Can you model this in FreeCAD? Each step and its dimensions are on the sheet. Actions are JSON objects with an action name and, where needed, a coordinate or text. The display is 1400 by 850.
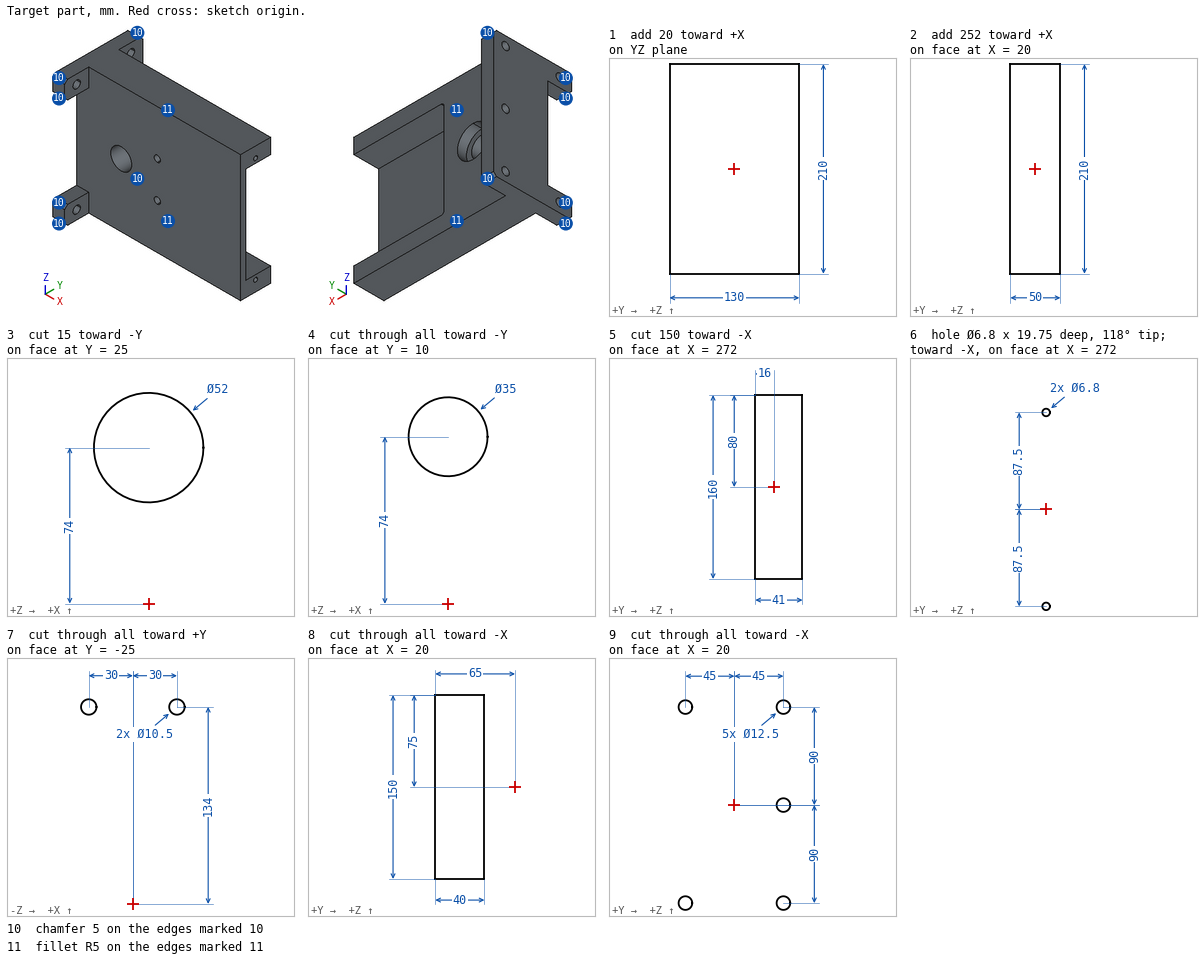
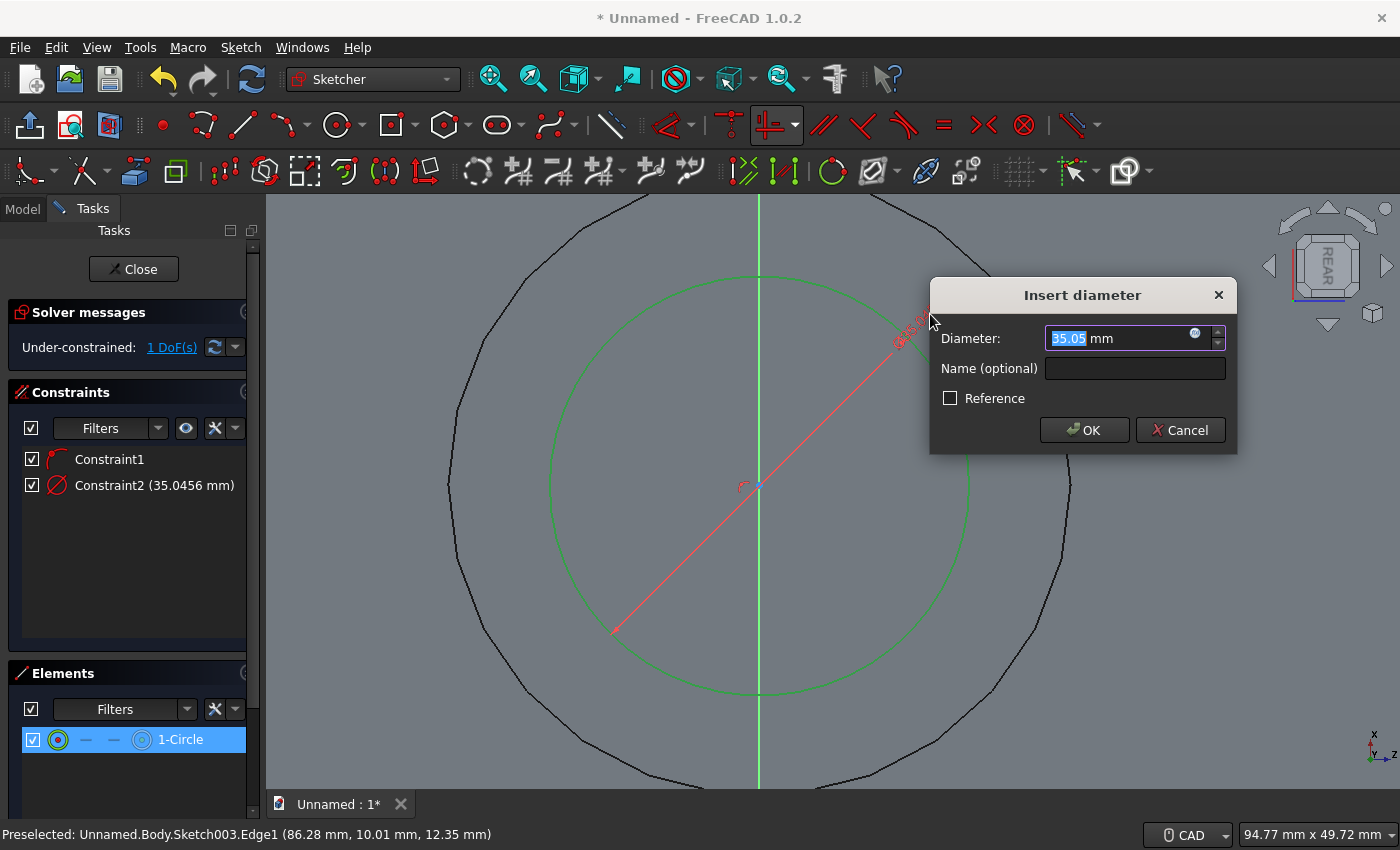
{"action": "type", "text": "35"}
{"action": "key", "text": "Return"}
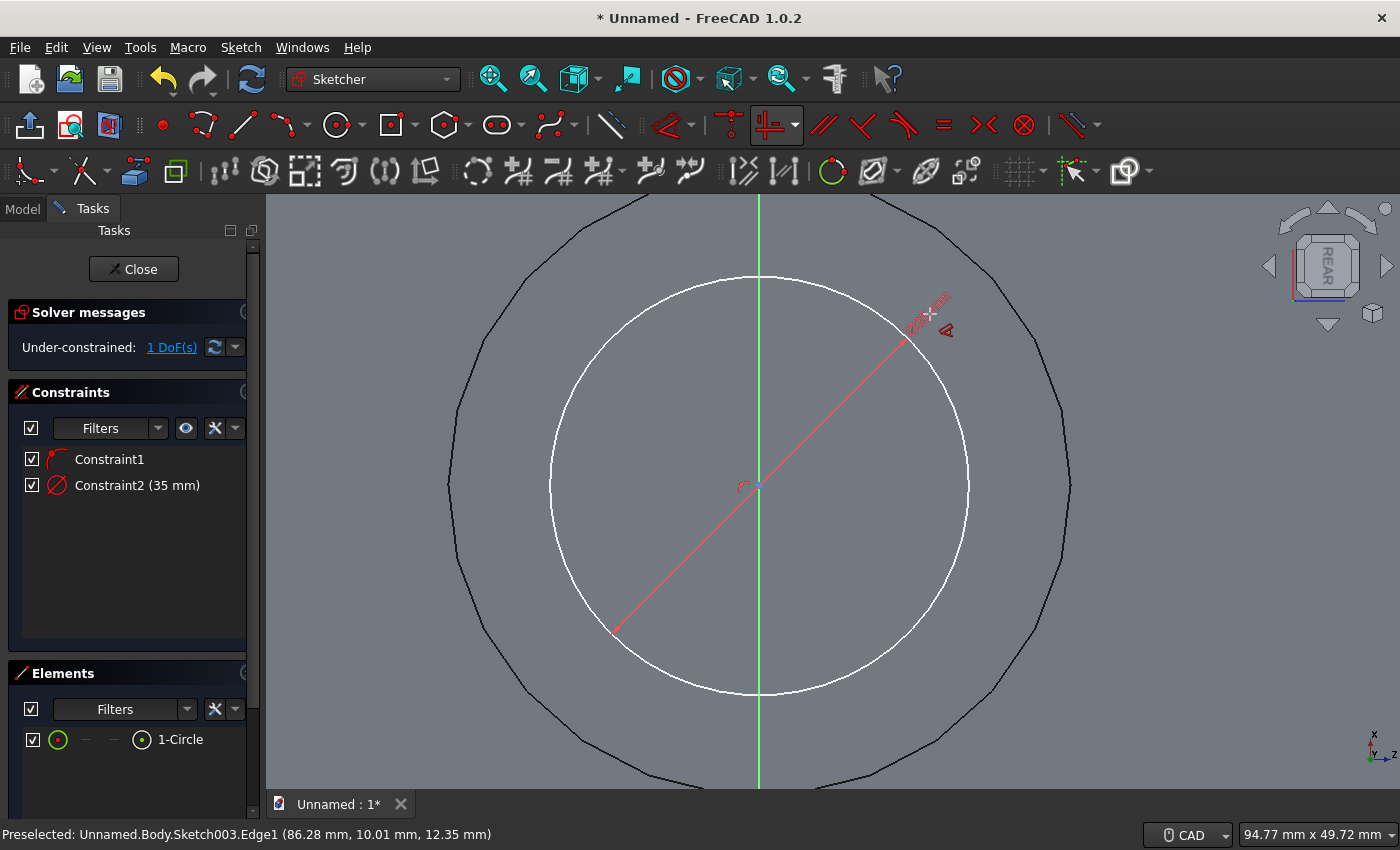
{"action": "left_click", "coordinate": [759, 486]}
{"action": "left_click", "coordinate": [793, 624]}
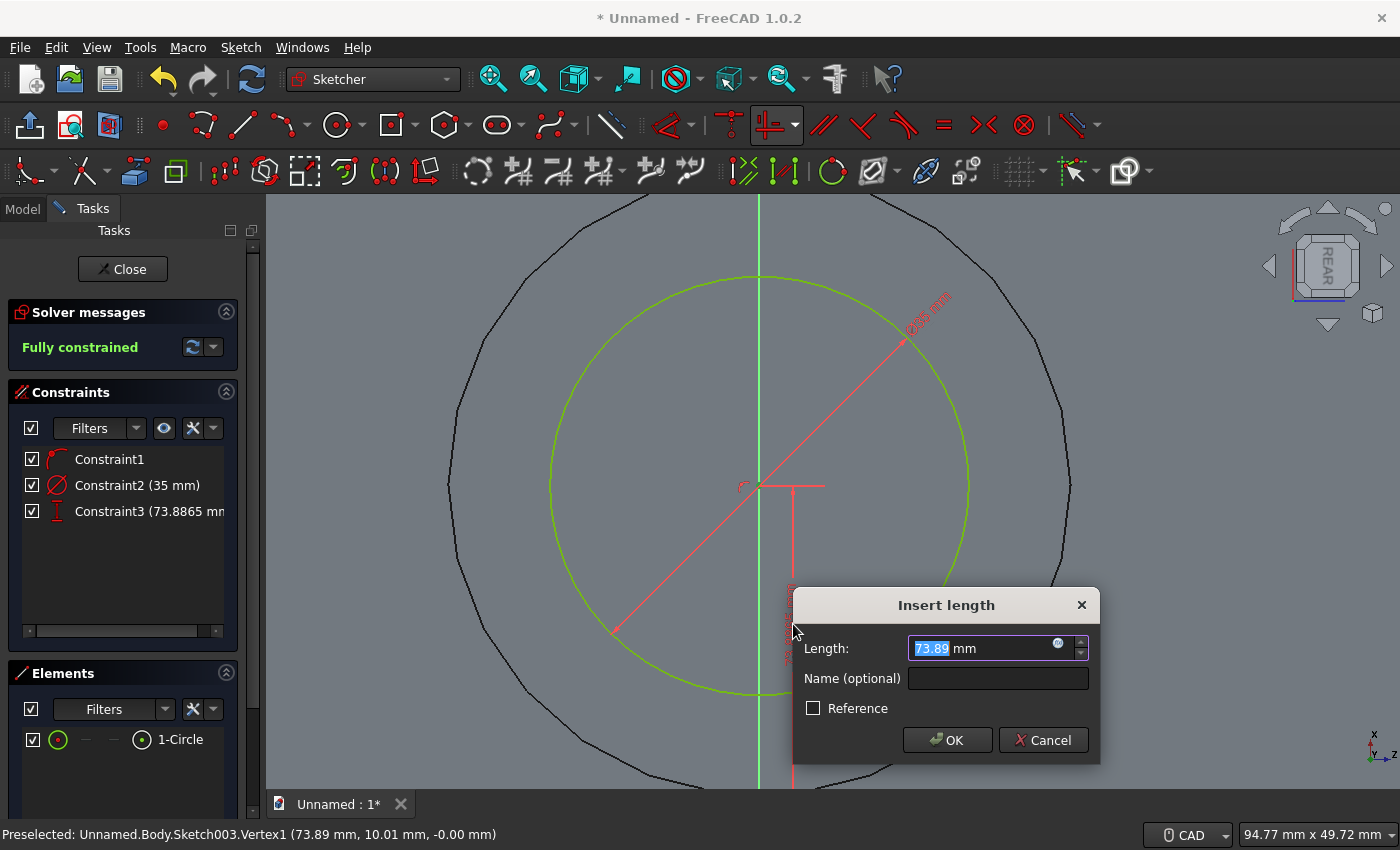
{"action": "type", "text": "74"}
{"action": "key", "text": "Return"}
{"action": "key", "text": "Escape"}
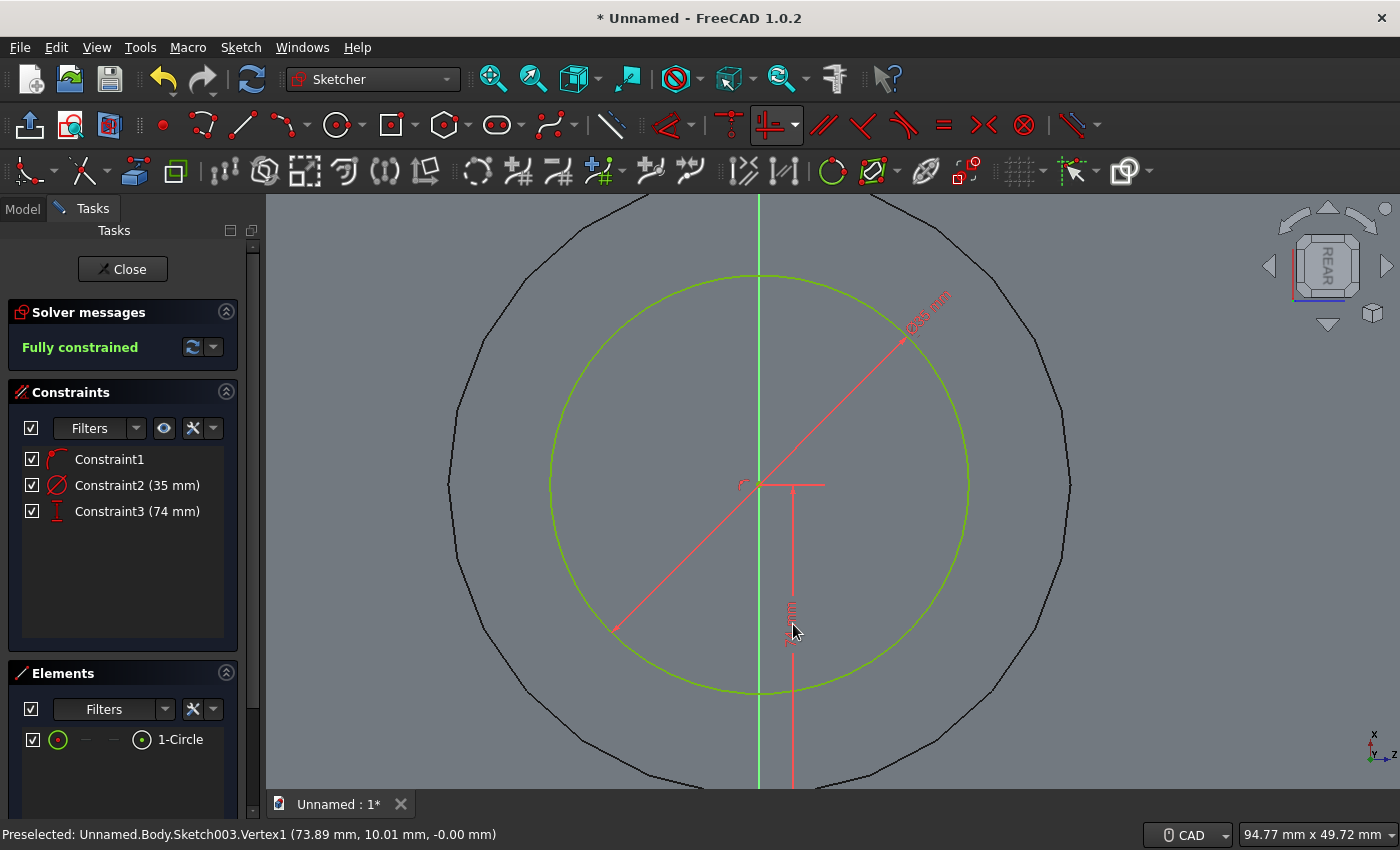
{"action": "left_click", "coordinate": [123, 269]}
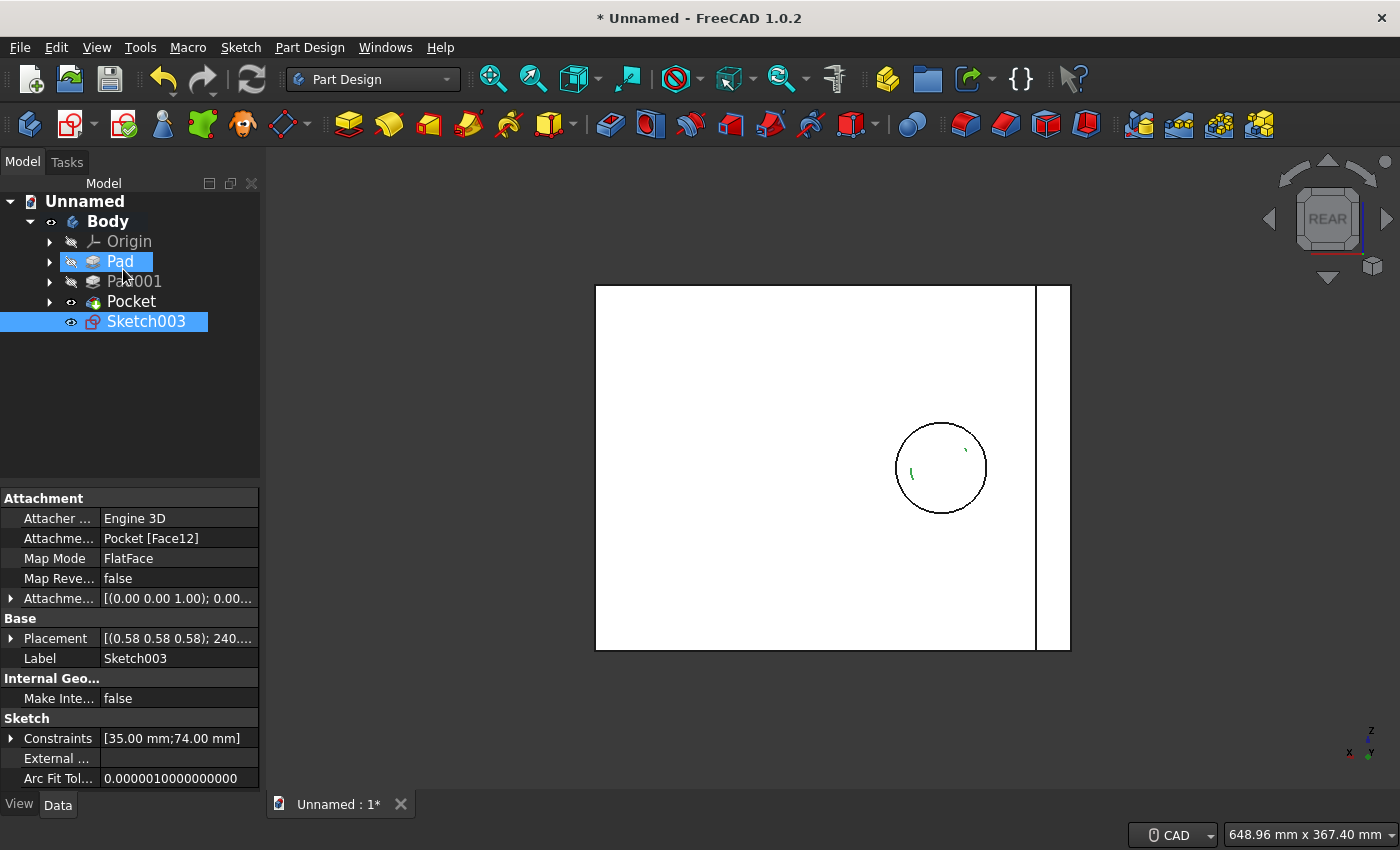
{"action": "left_click", "coordinate": [612, 124]}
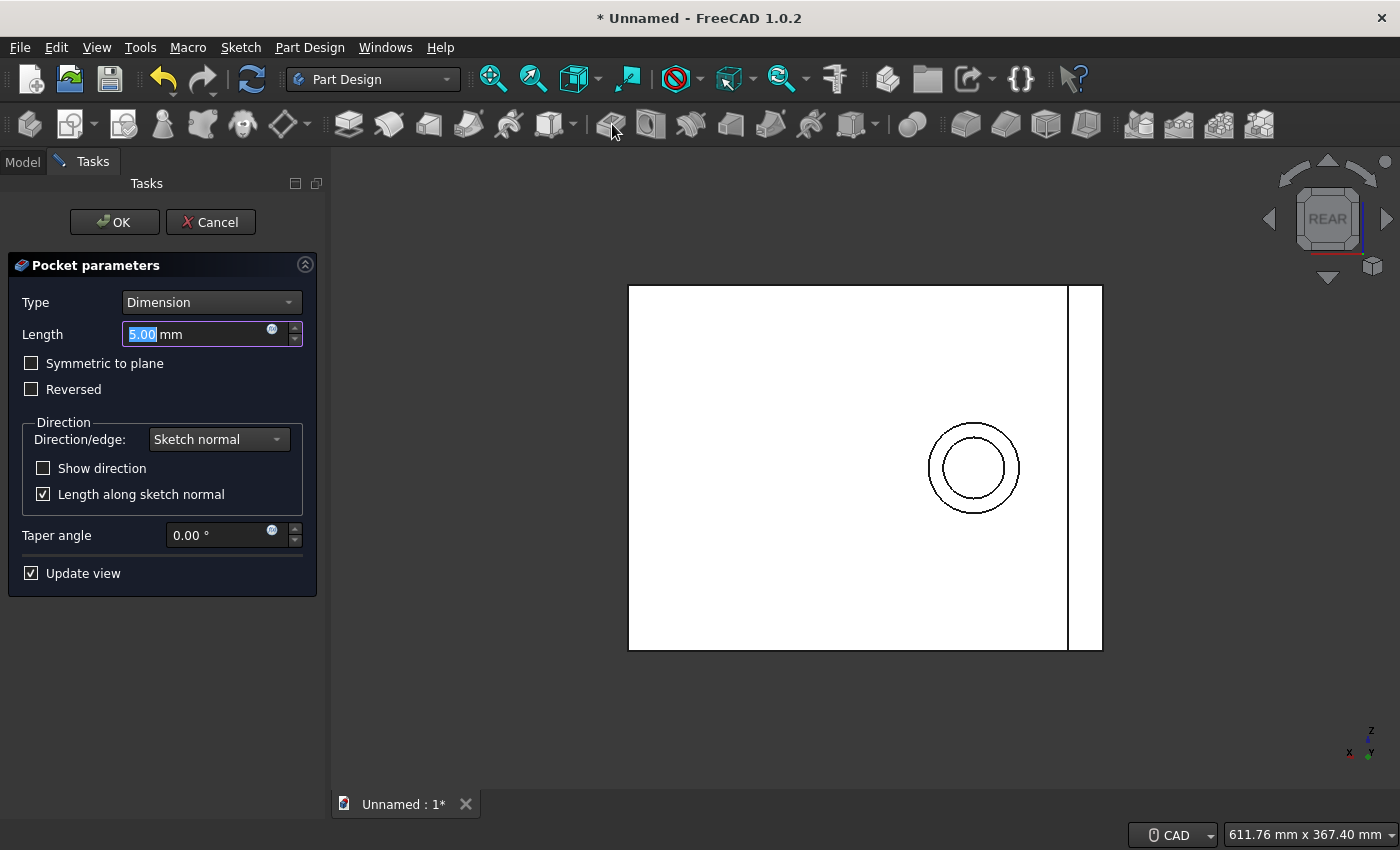
{"action": "left_click", "coordinate": [212, 302]}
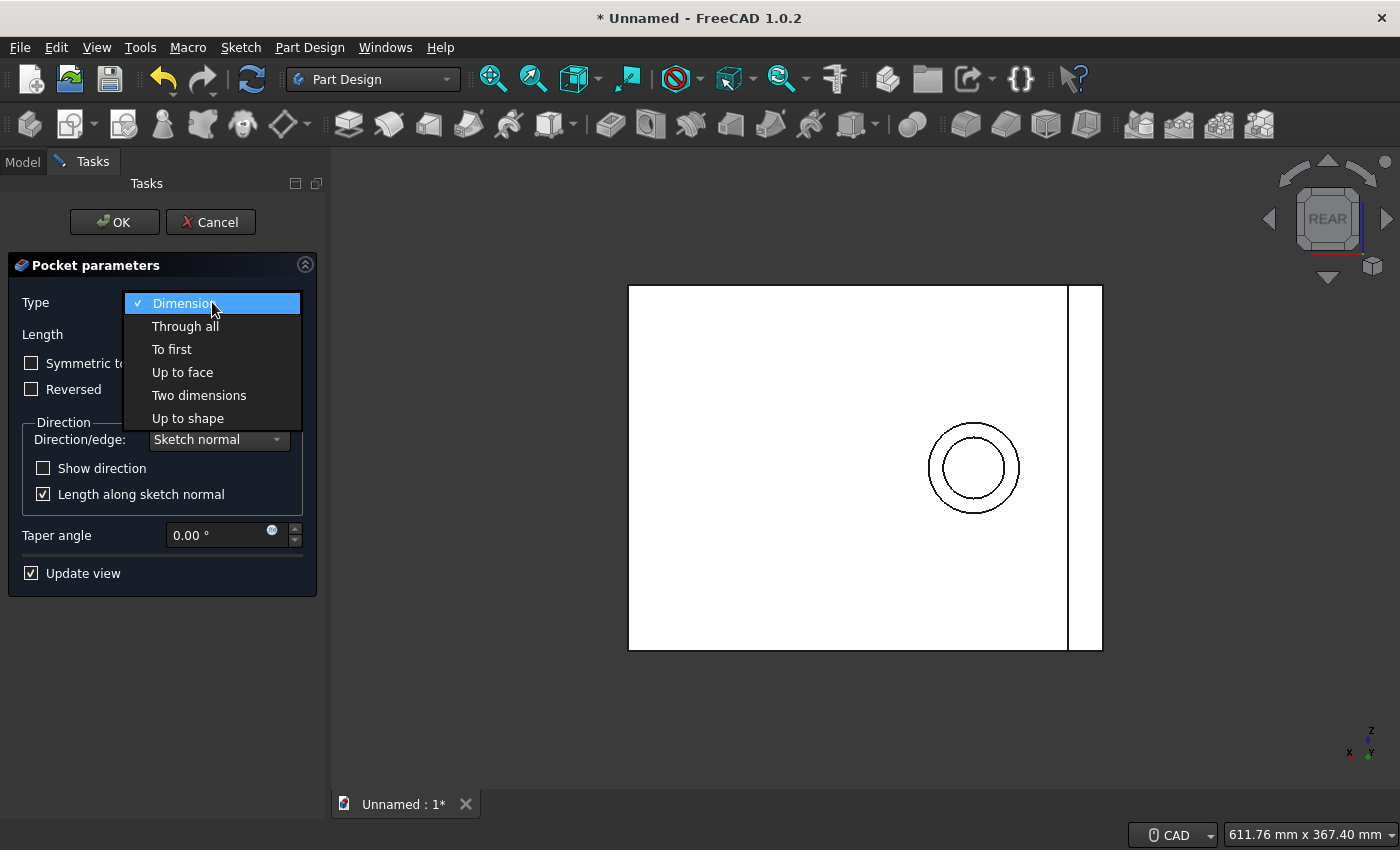
{"action": "left_click", "coordinate": [212, 326]}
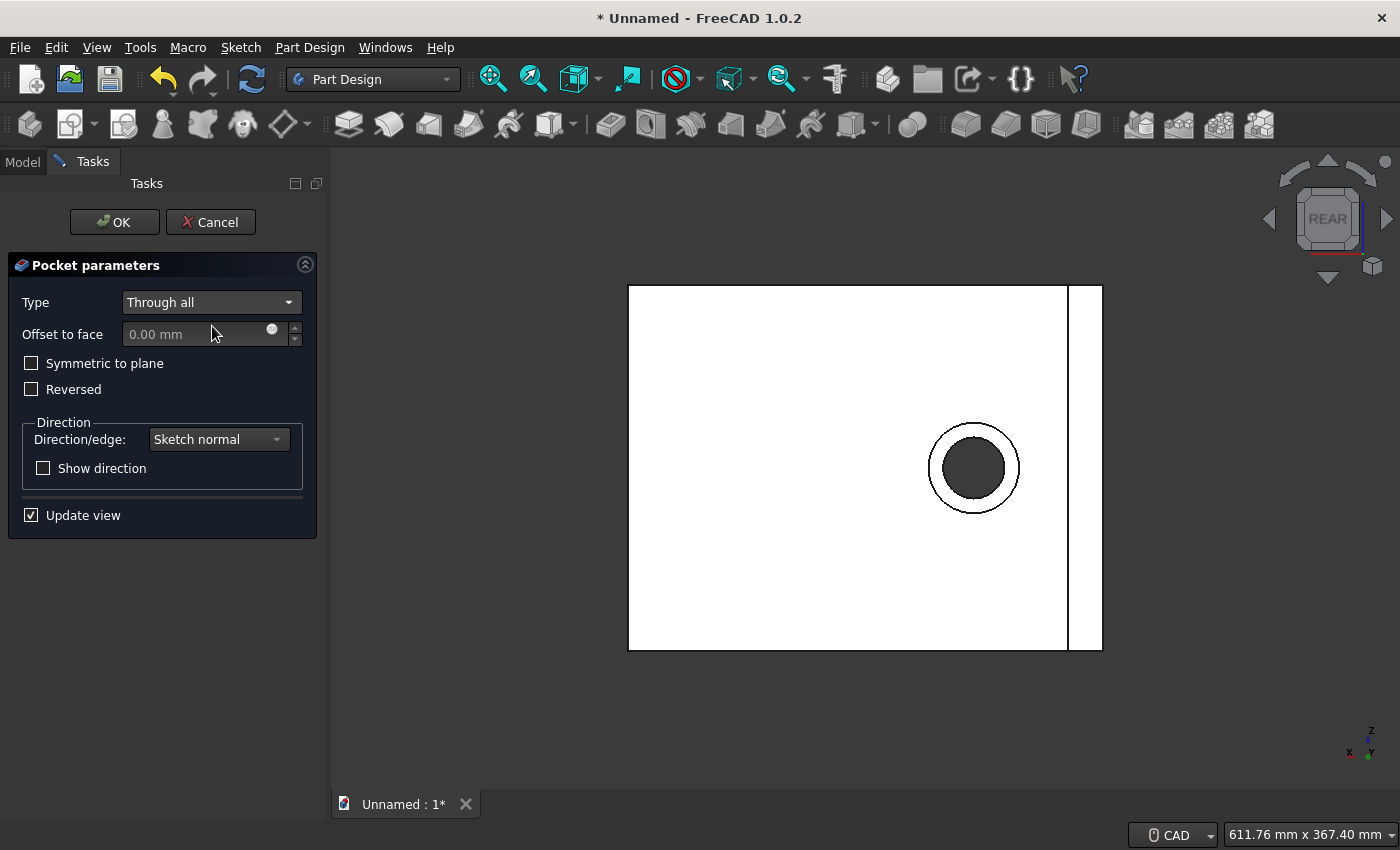
{"action": "left_click", "coordinate": [115, 222]}